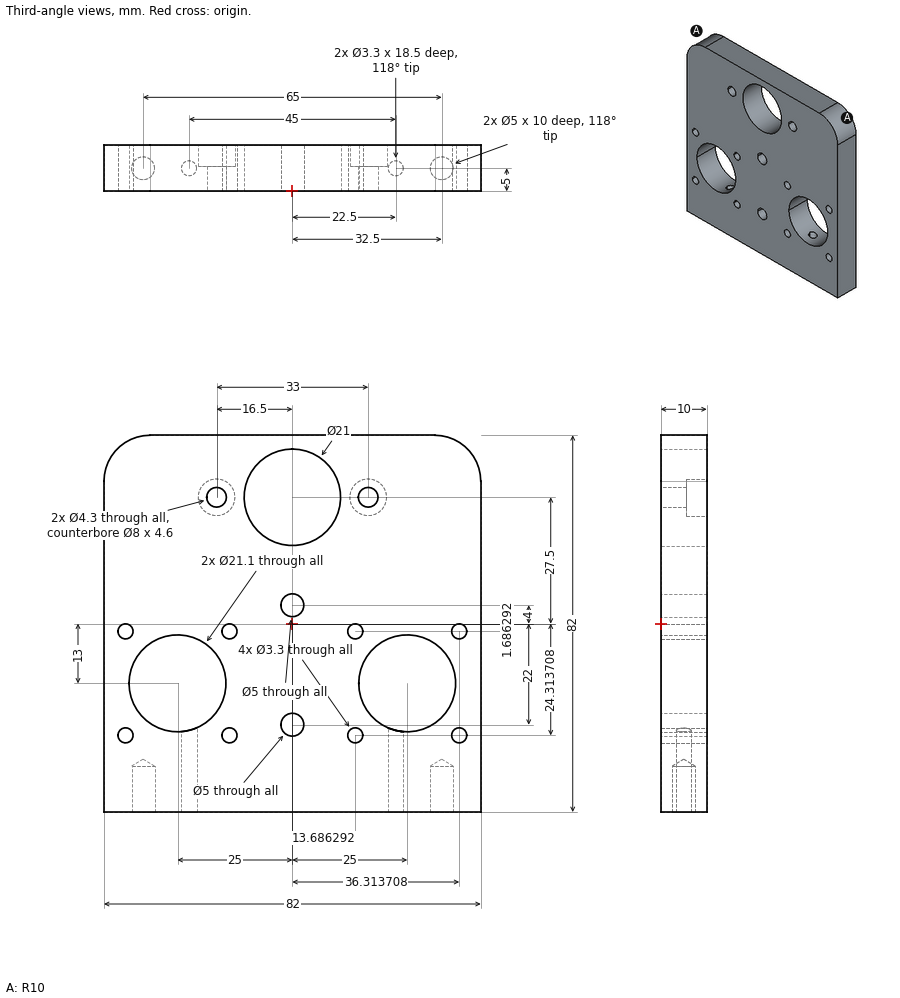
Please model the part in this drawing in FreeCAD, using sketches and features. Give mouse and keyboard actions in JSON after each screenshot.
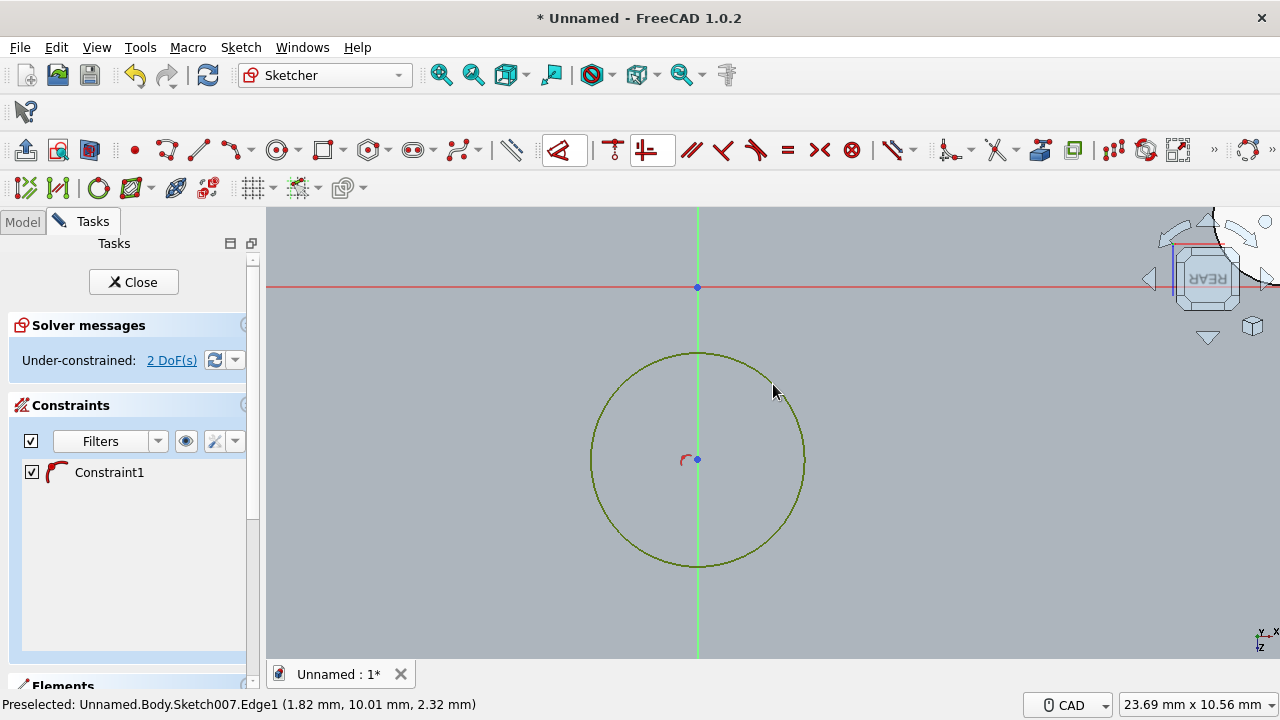
{"action": "left_click", "coordinate": [582, 150]}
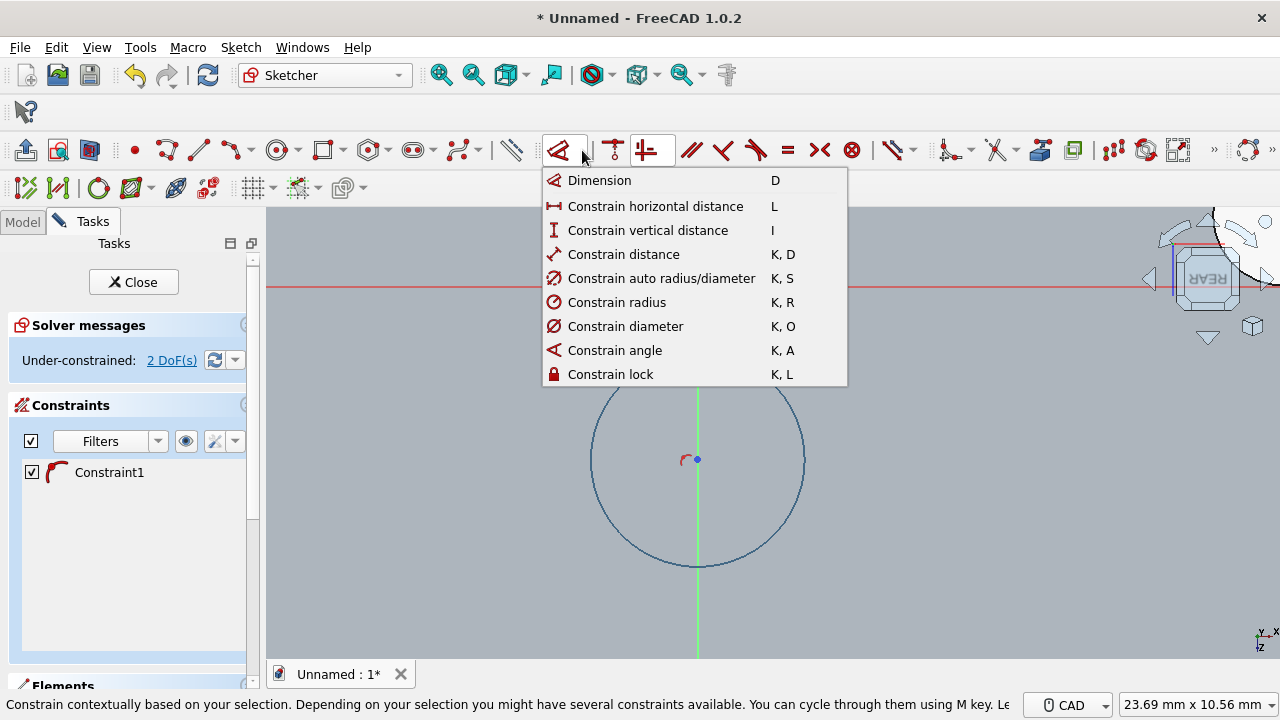
{"action": "left_click", "coordinate": [695, 326]}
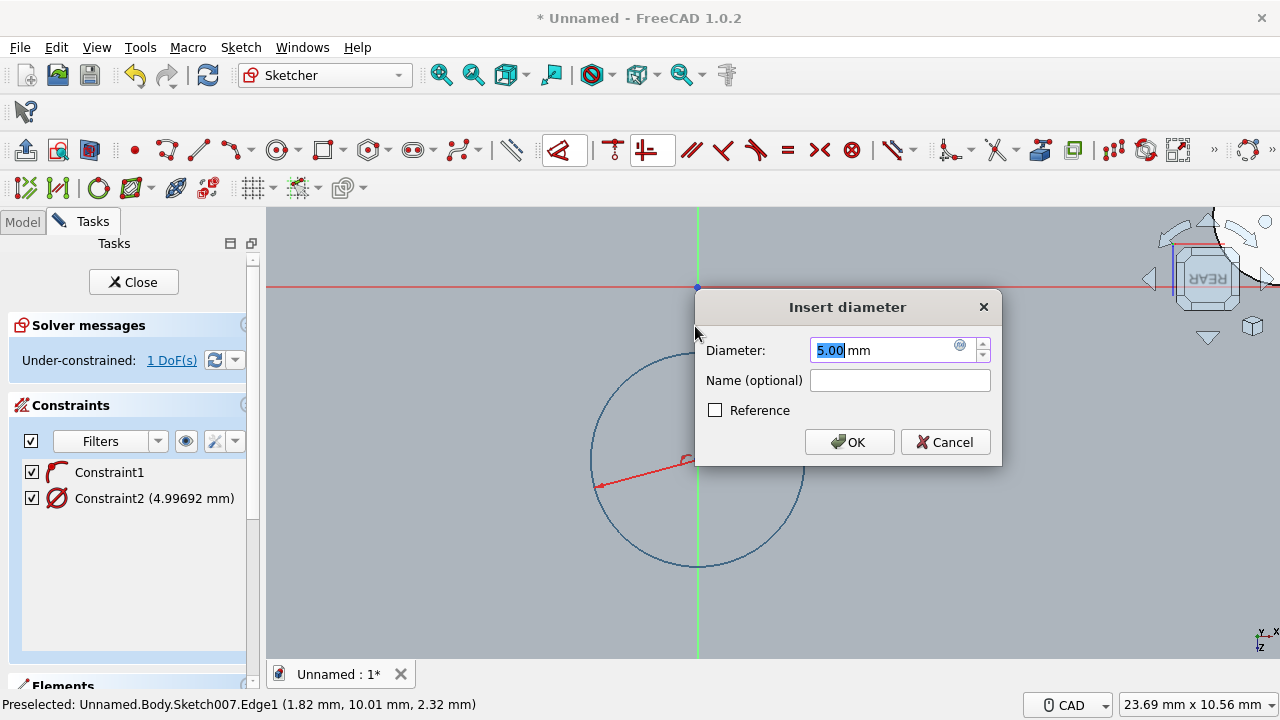
{"action": "type", "text": "5"}
{"action": "key", "text": "Return"}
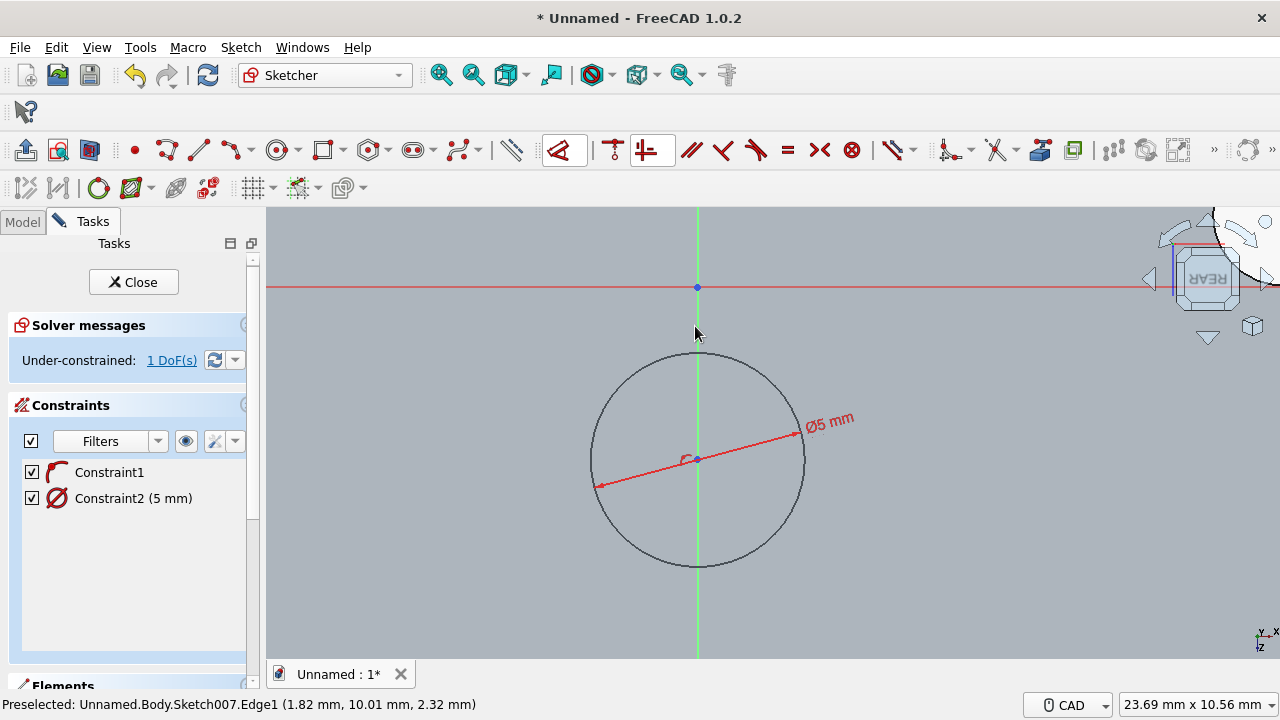
{"action": "left_click", "coordinate": [698, 460]}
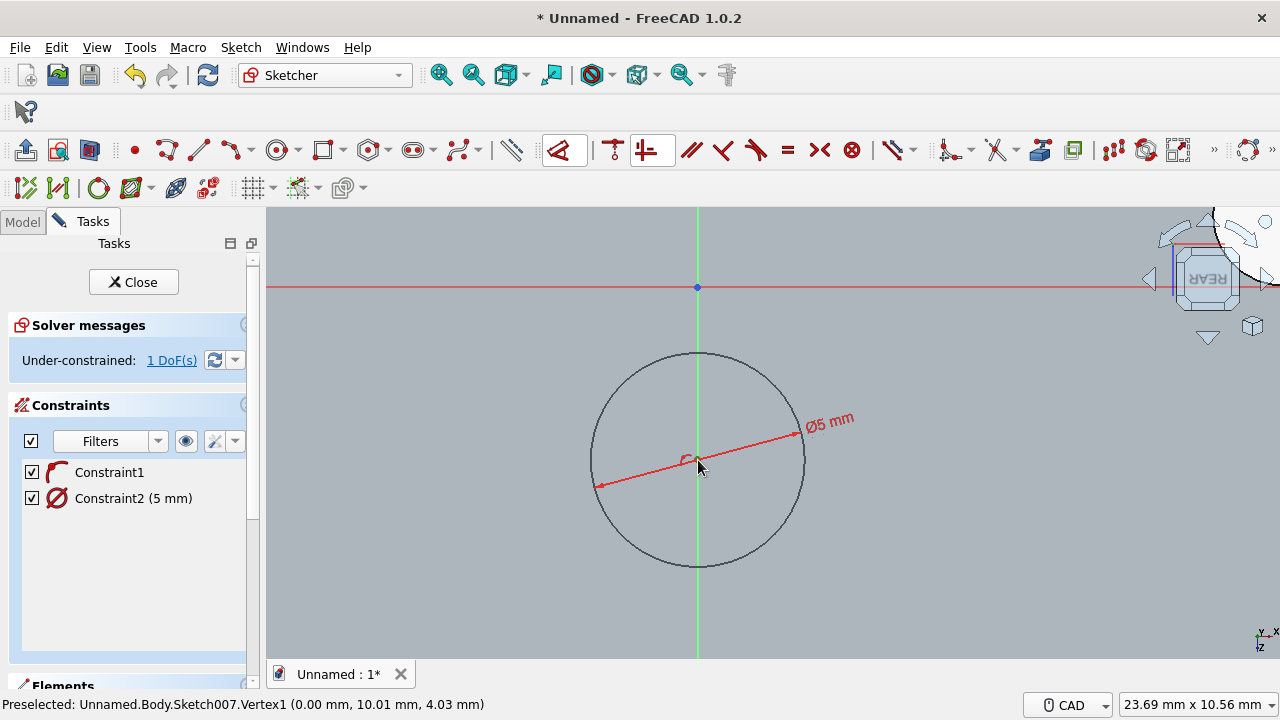
{"action": "key", "text": "i"}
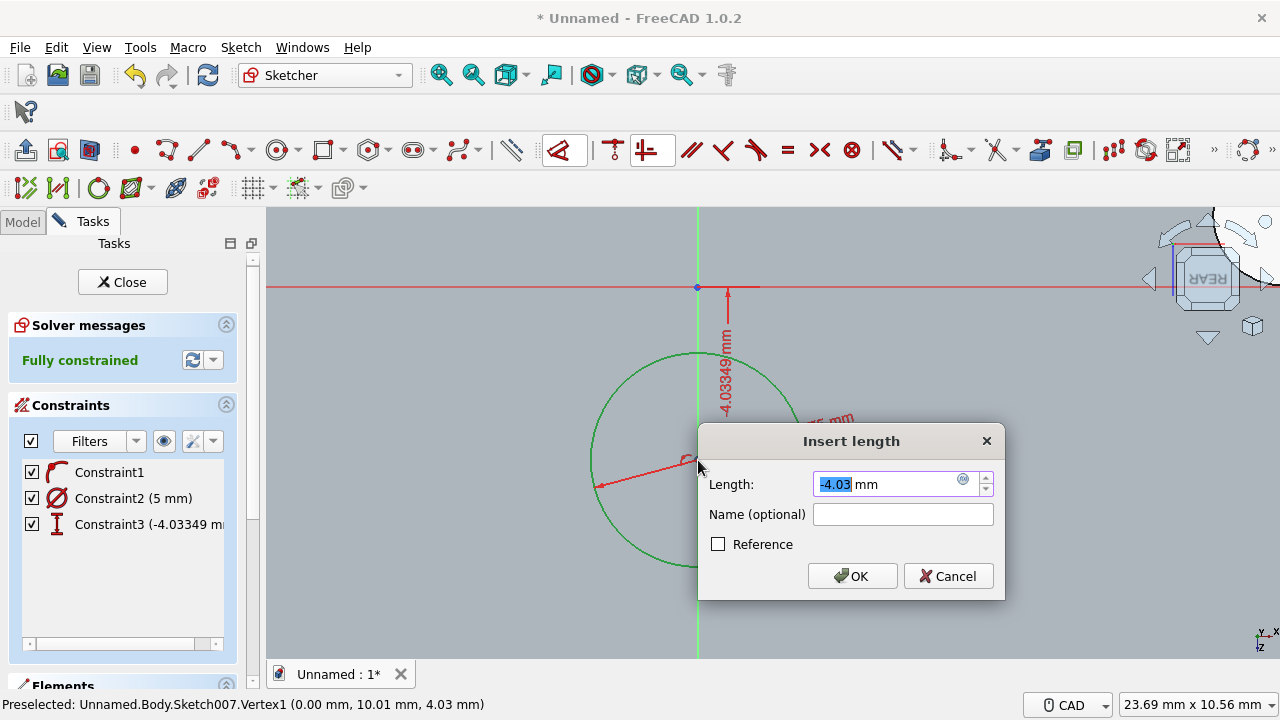
{"action": "type", "text": "-4"}
{"action": "key", "text": "Return"}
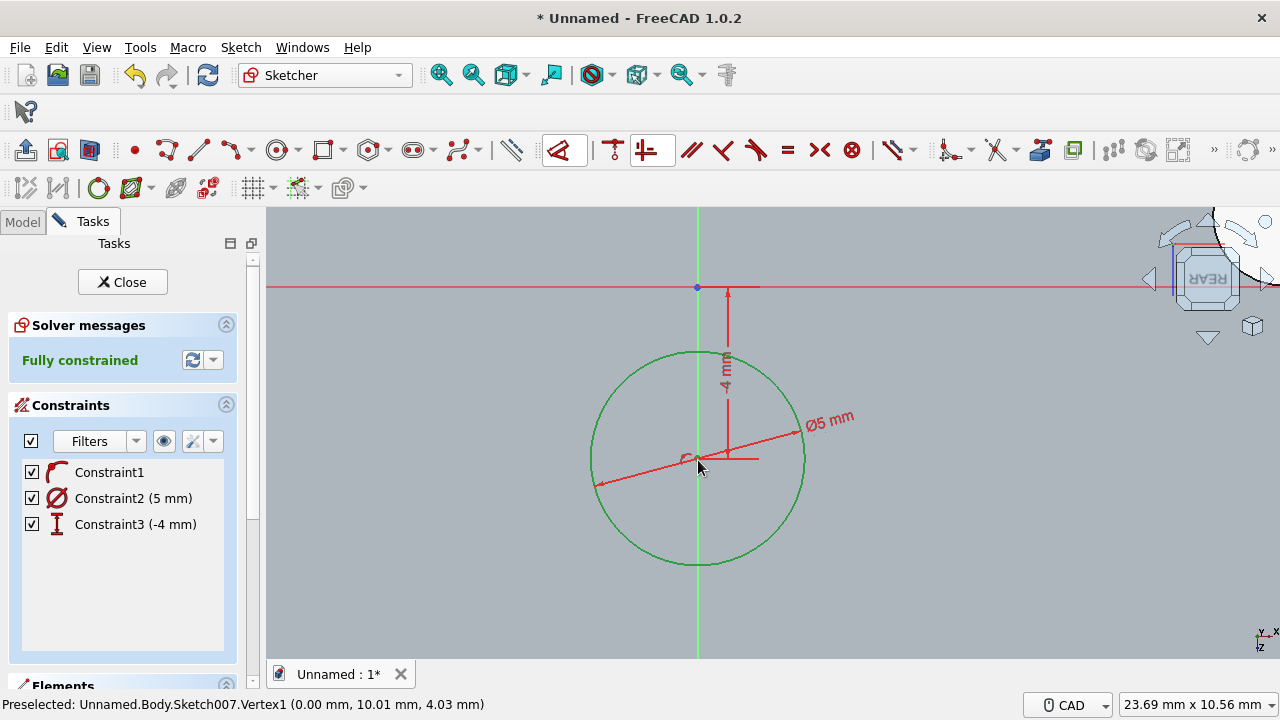
{"action": "left_click", "coordinate": [123, 282]}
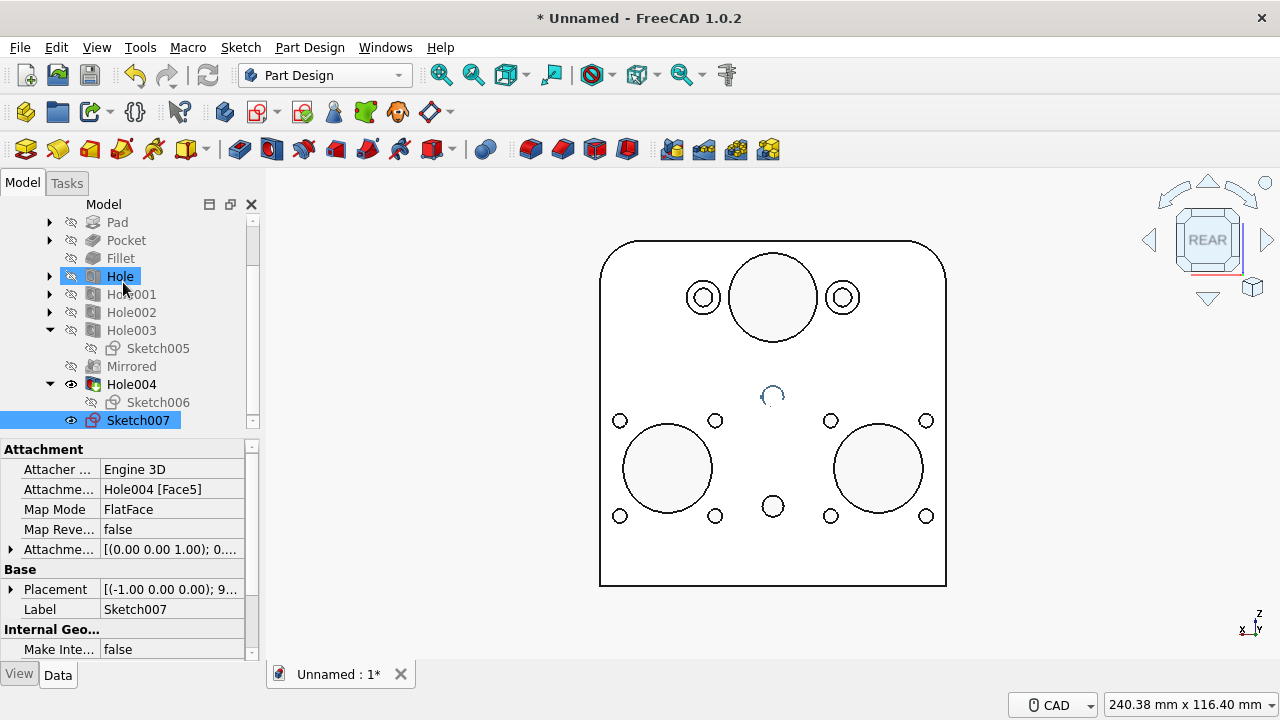
{"action": "left_click", "coordinate": [272, 150]}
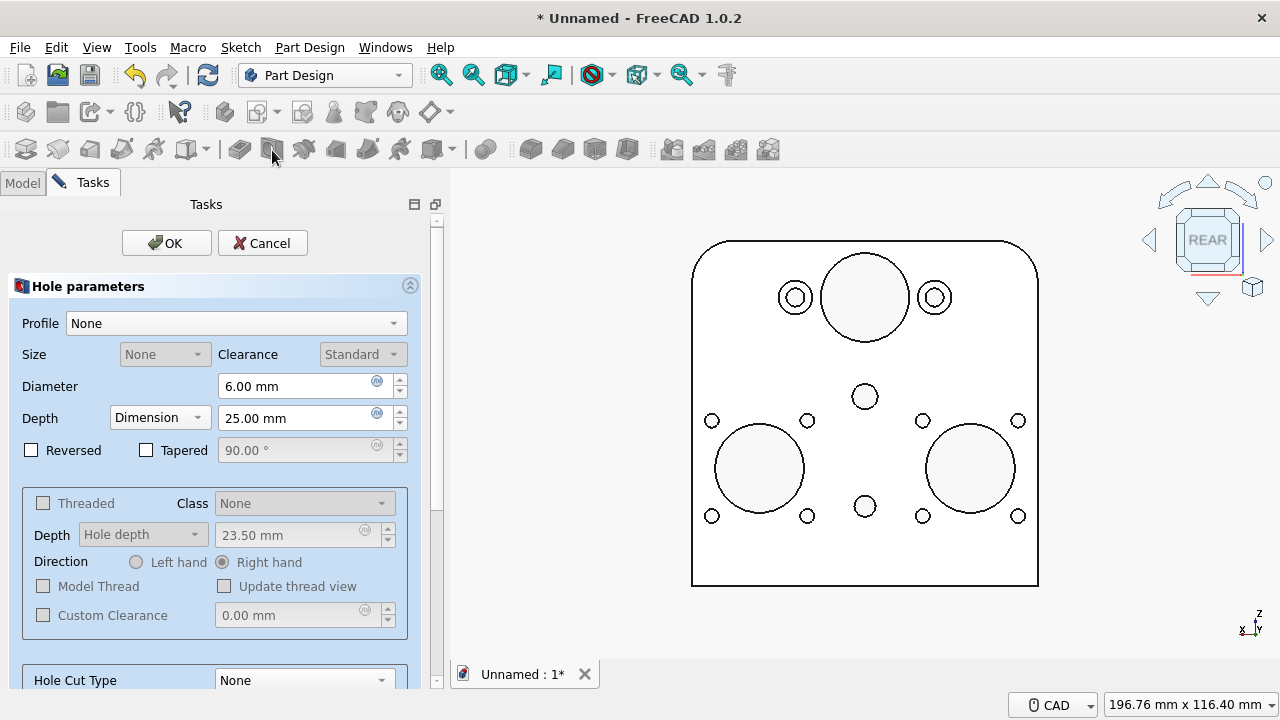
{"action": "triple_click", "coordinate": [305, 386]}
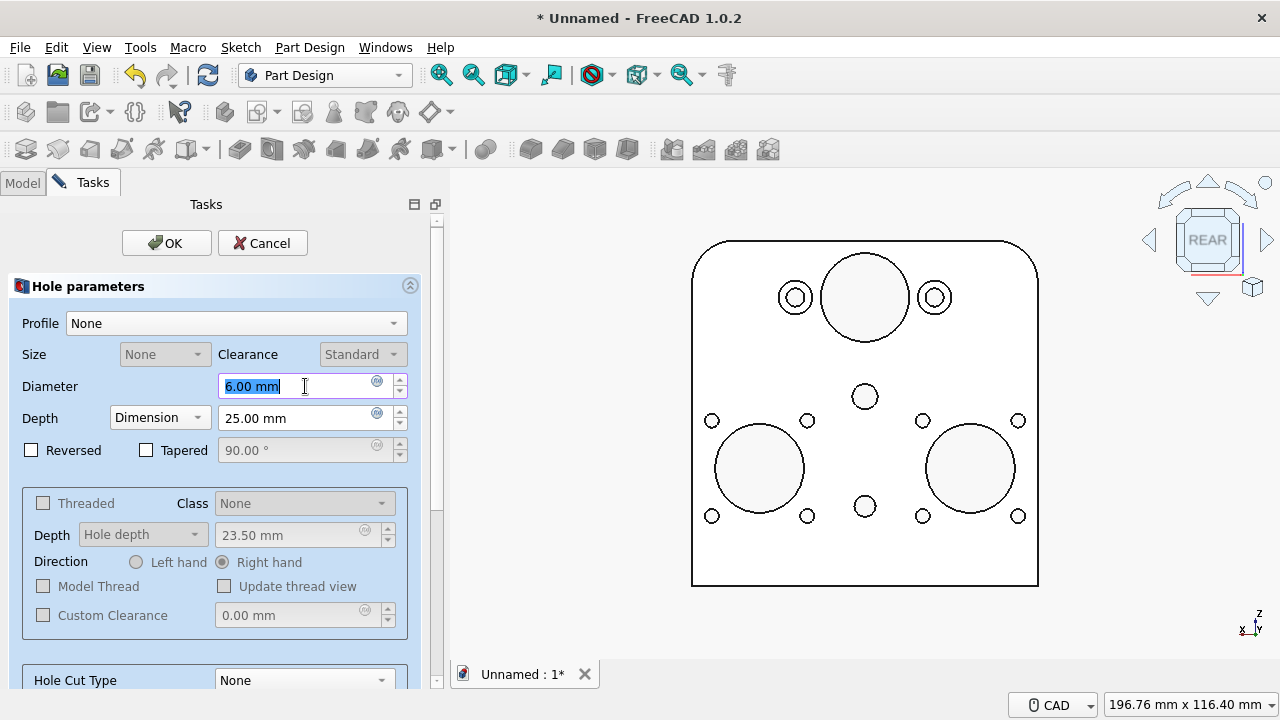
{"action": "type", "text": "5"}
{"action": "key", "text": "Tab"}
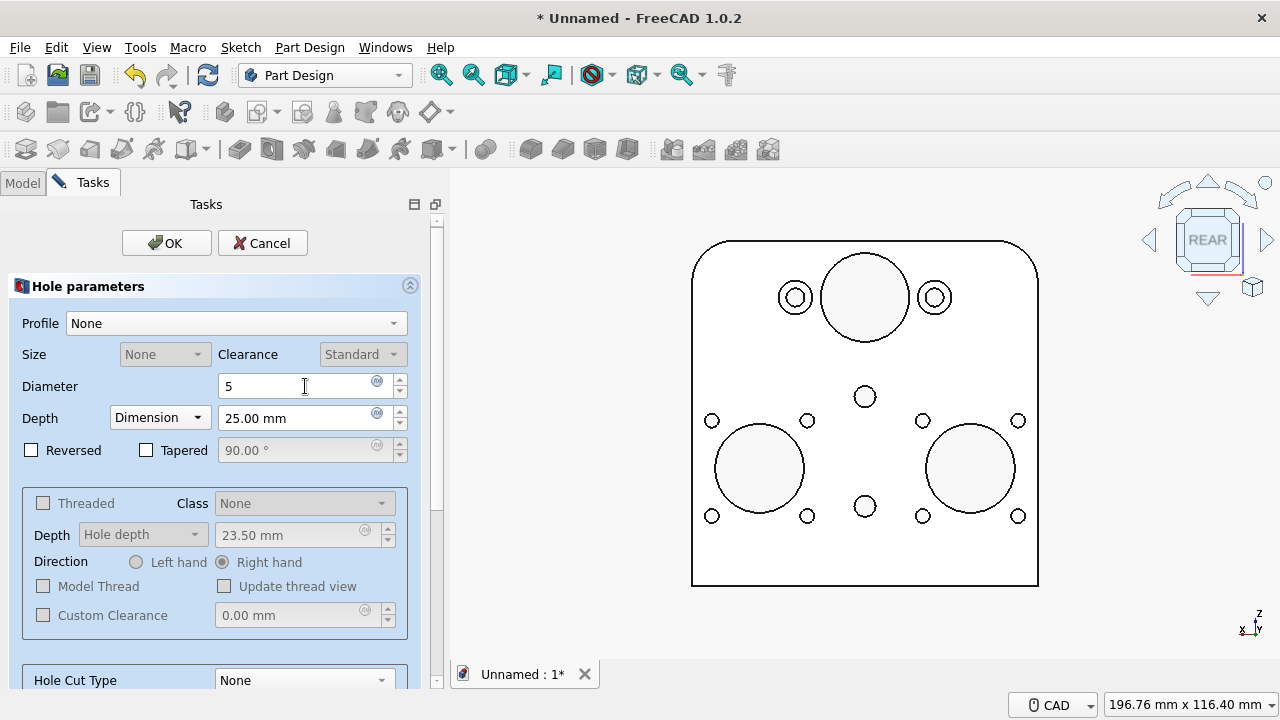
{"action": "left_click", "coordinate": [161, 418]}